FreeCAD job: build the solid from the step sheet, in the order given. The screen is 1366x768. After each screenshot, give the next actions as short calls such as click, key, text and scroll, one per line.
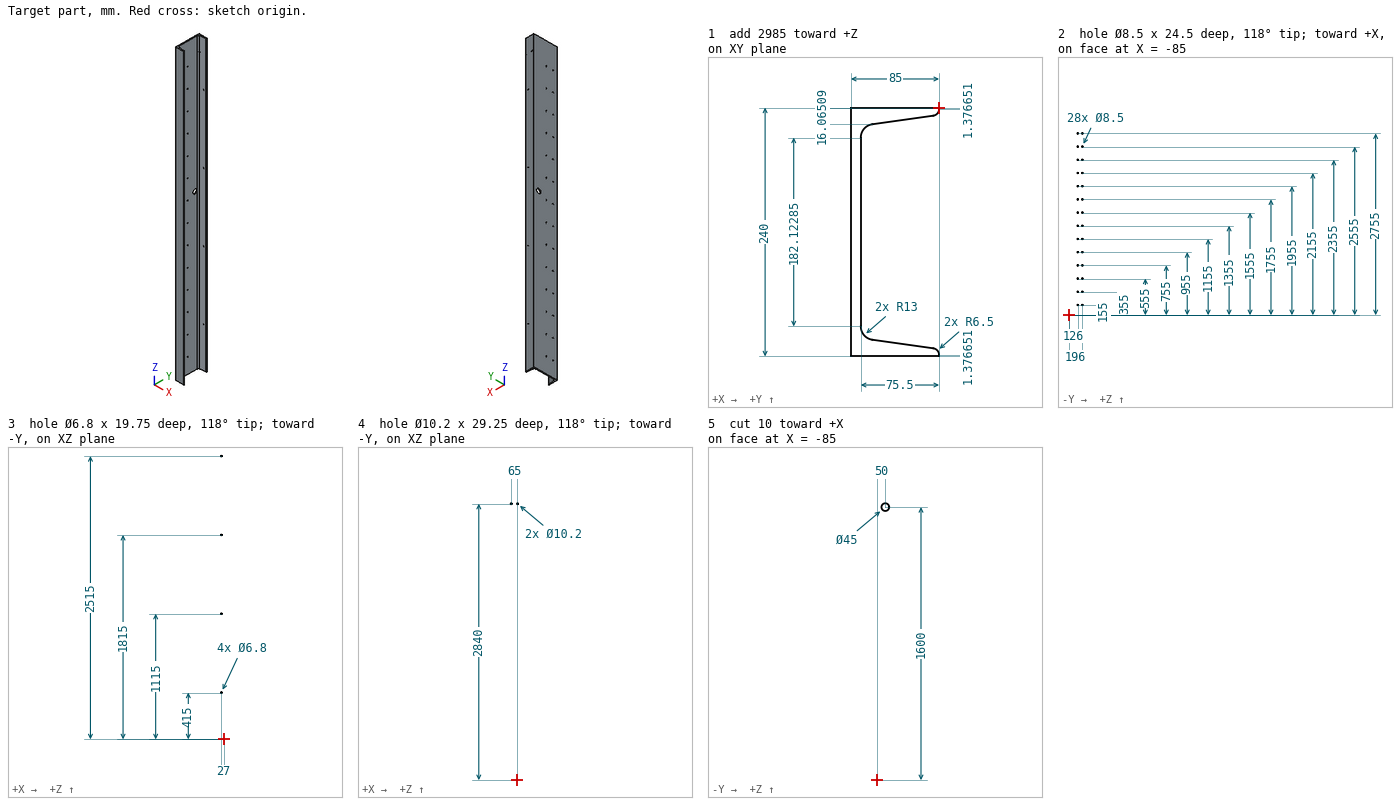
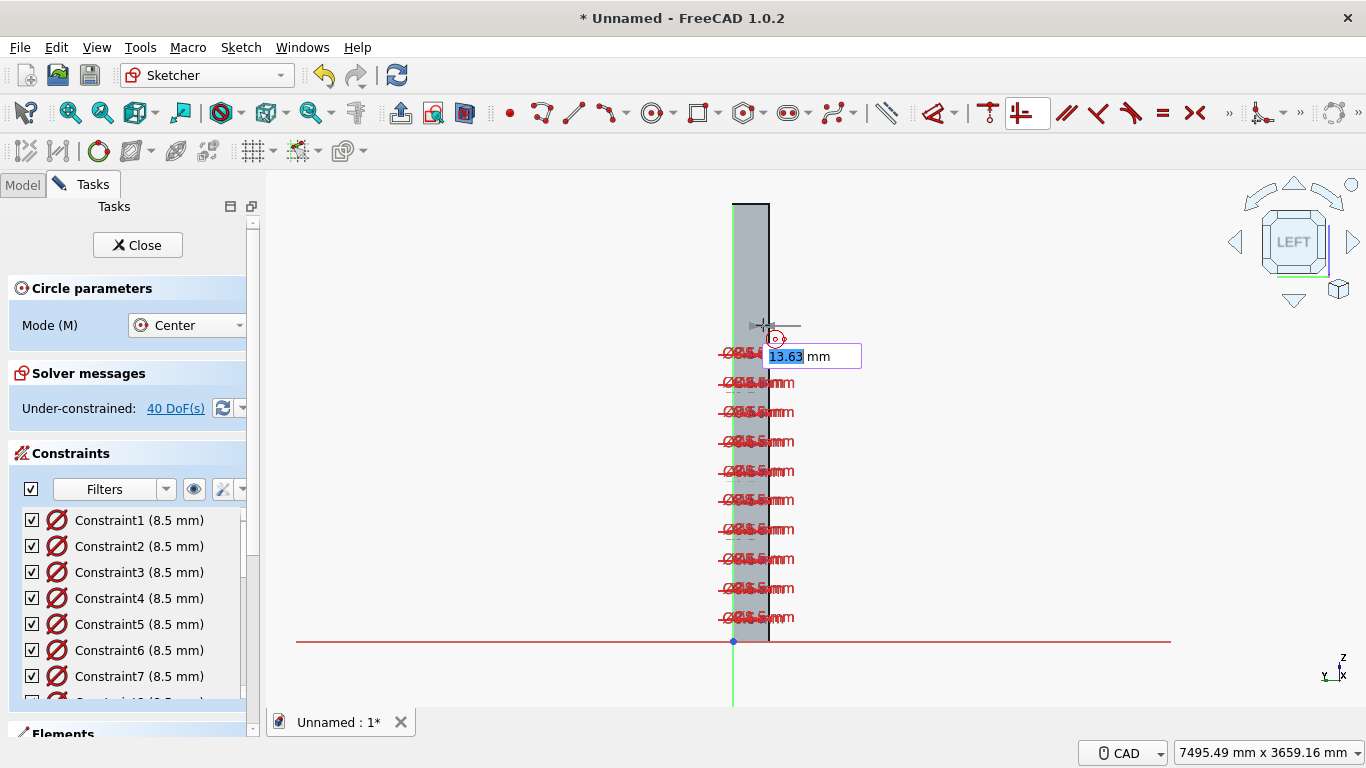
text(8.5)
key(Return)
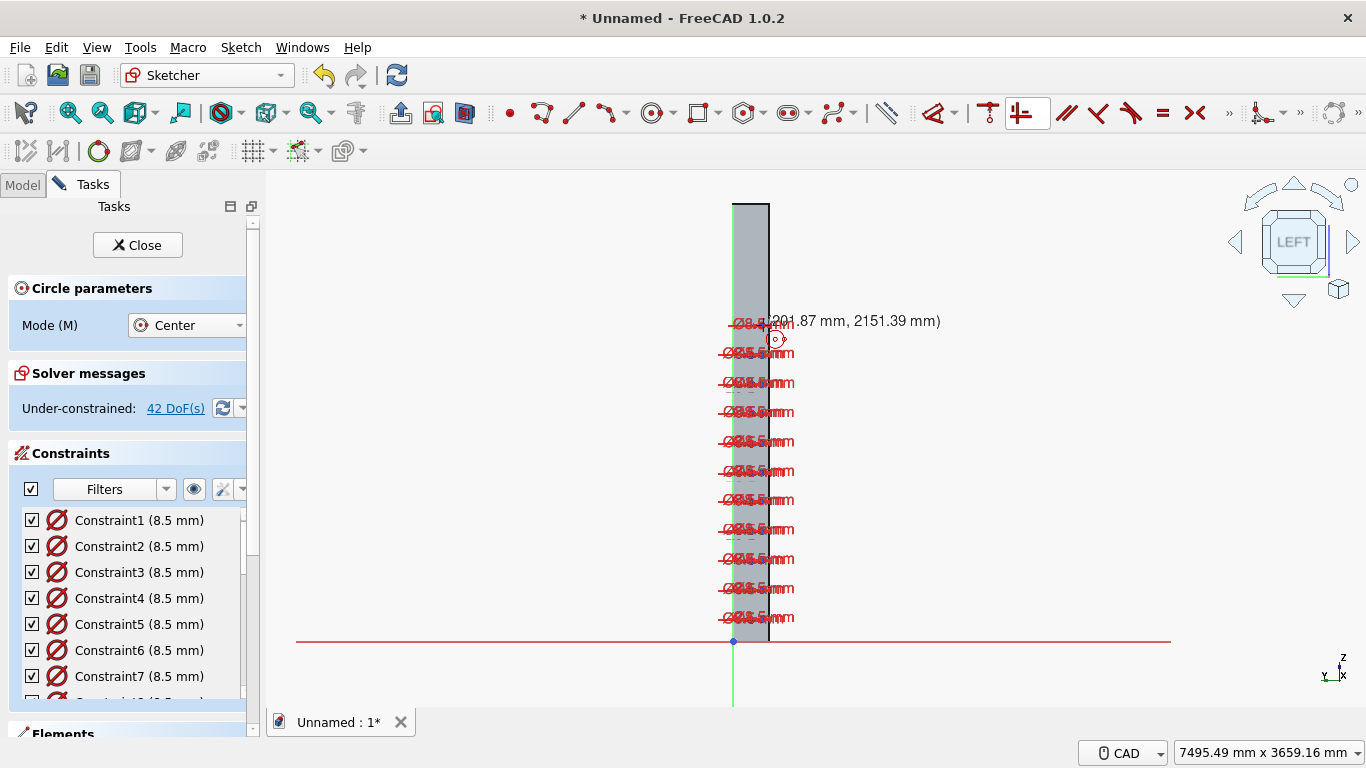
scroll(752, 325, up, 18)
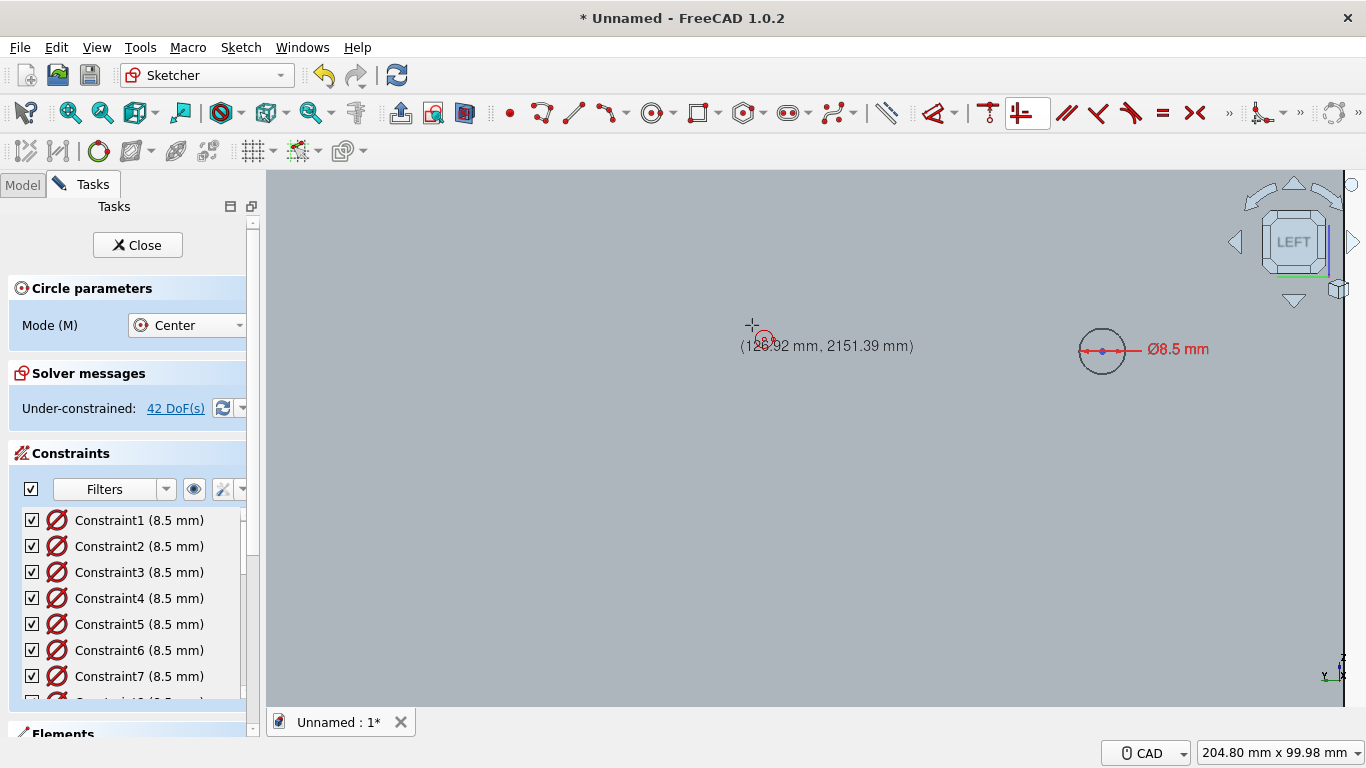
scroll(752, 325, down, 18)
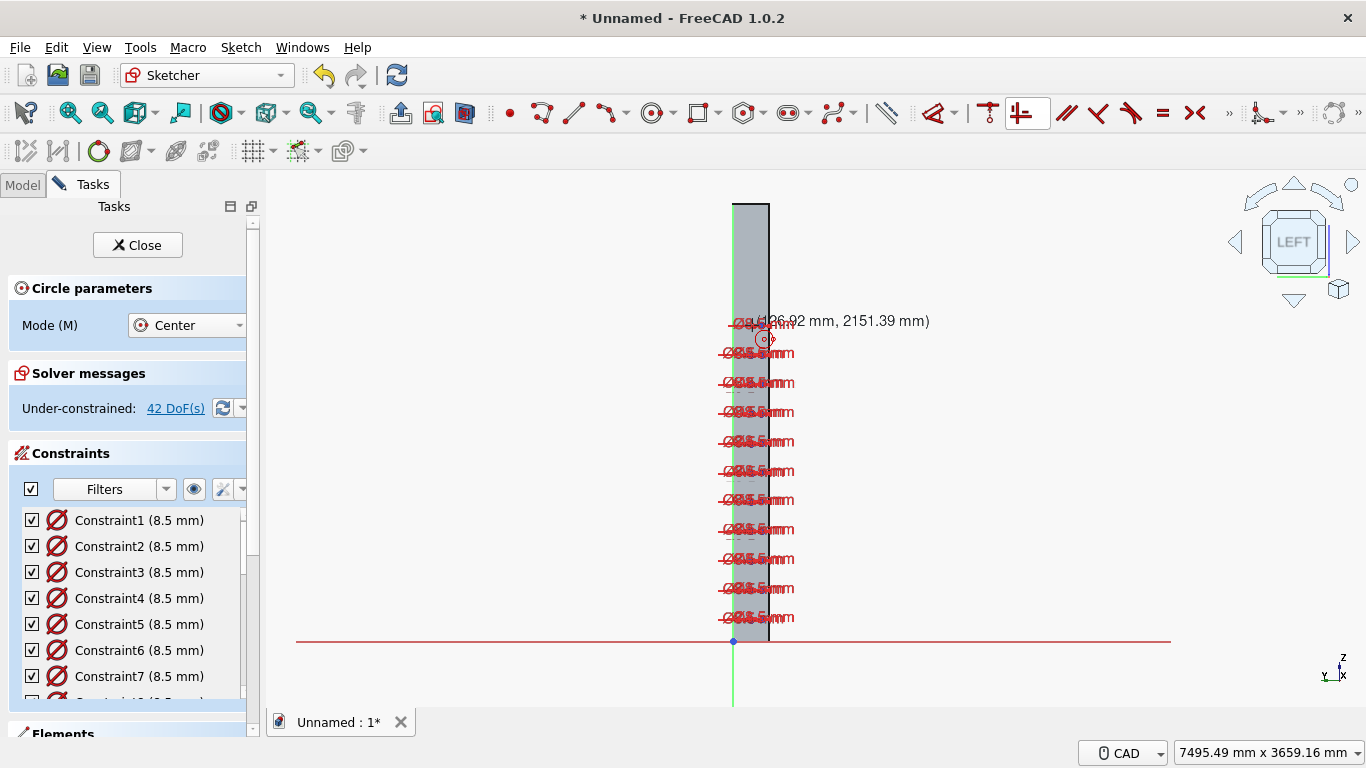
scroll(752, 325, up, 3)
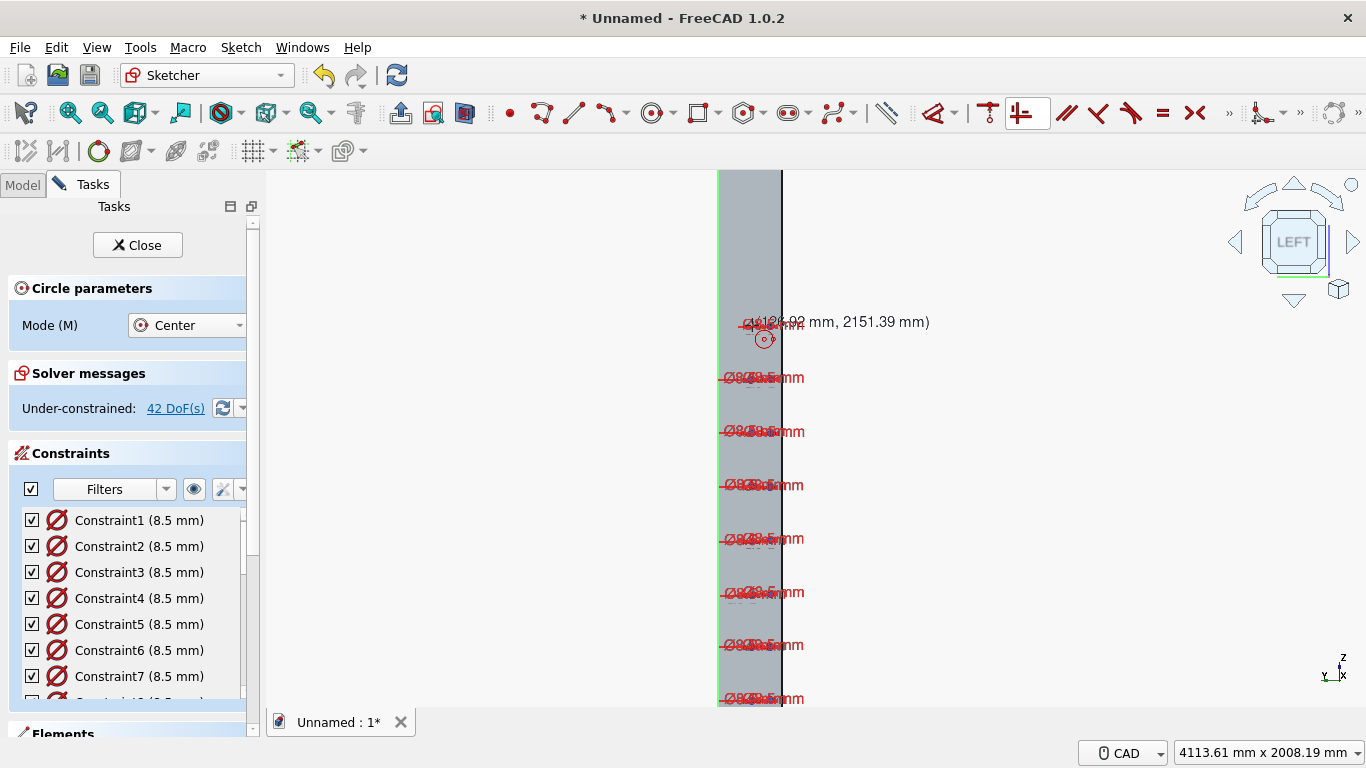
click(751, 326)
move(752, 325)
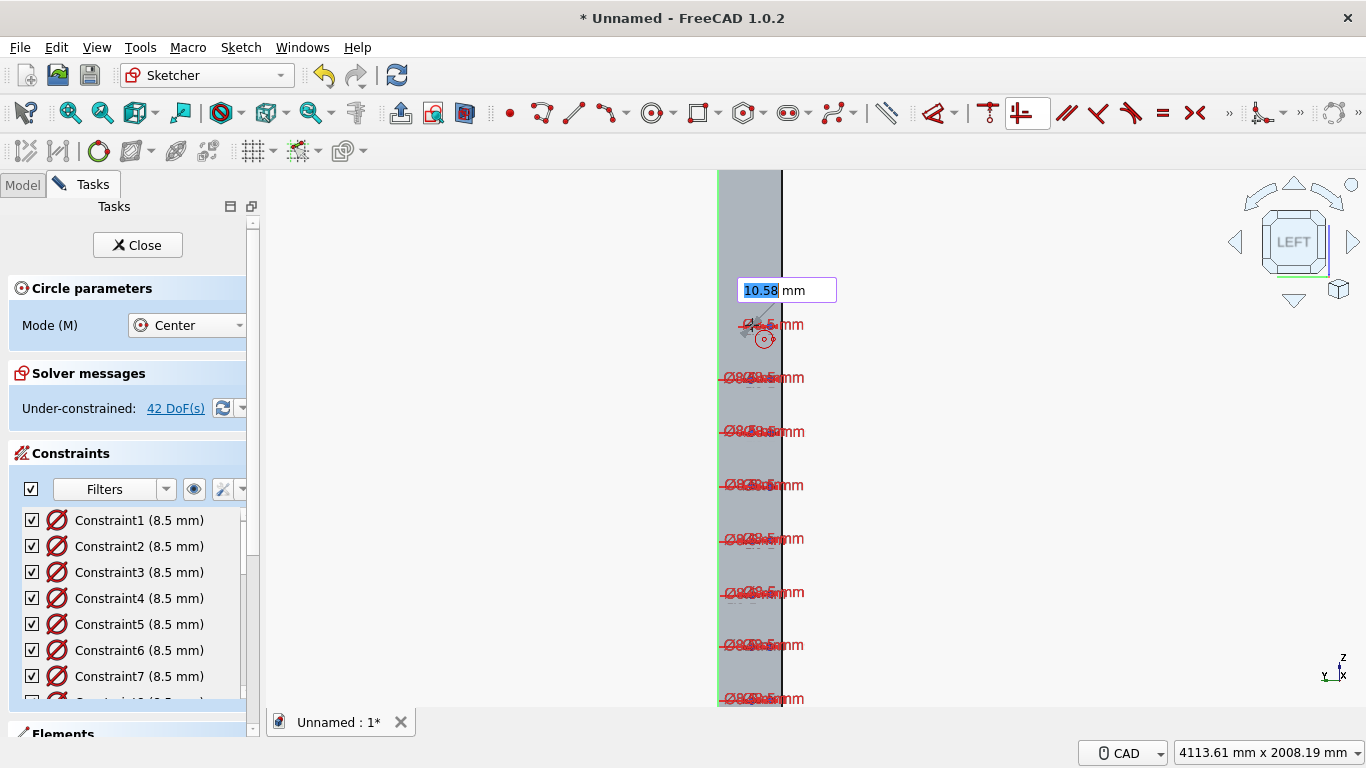
text(8.5)
key(Return)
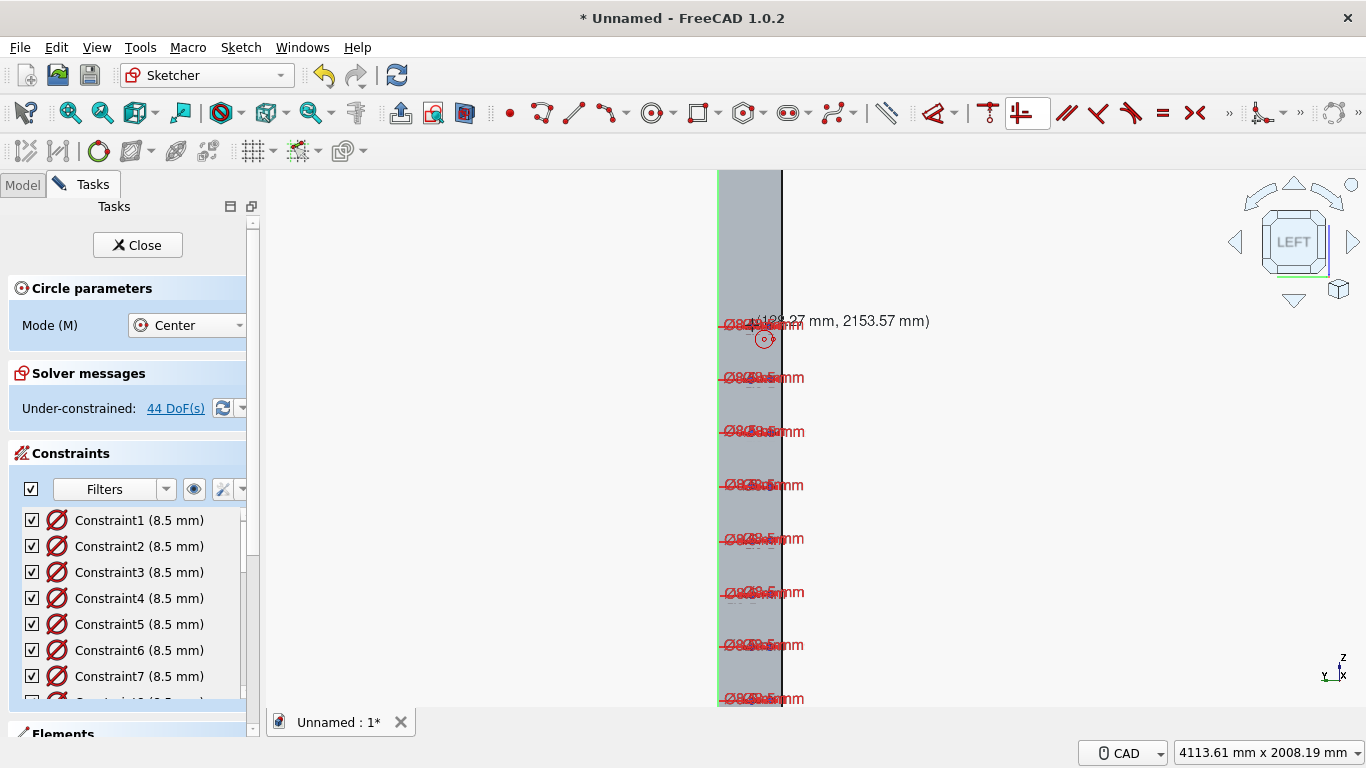
scroll(751, 272, up, 15)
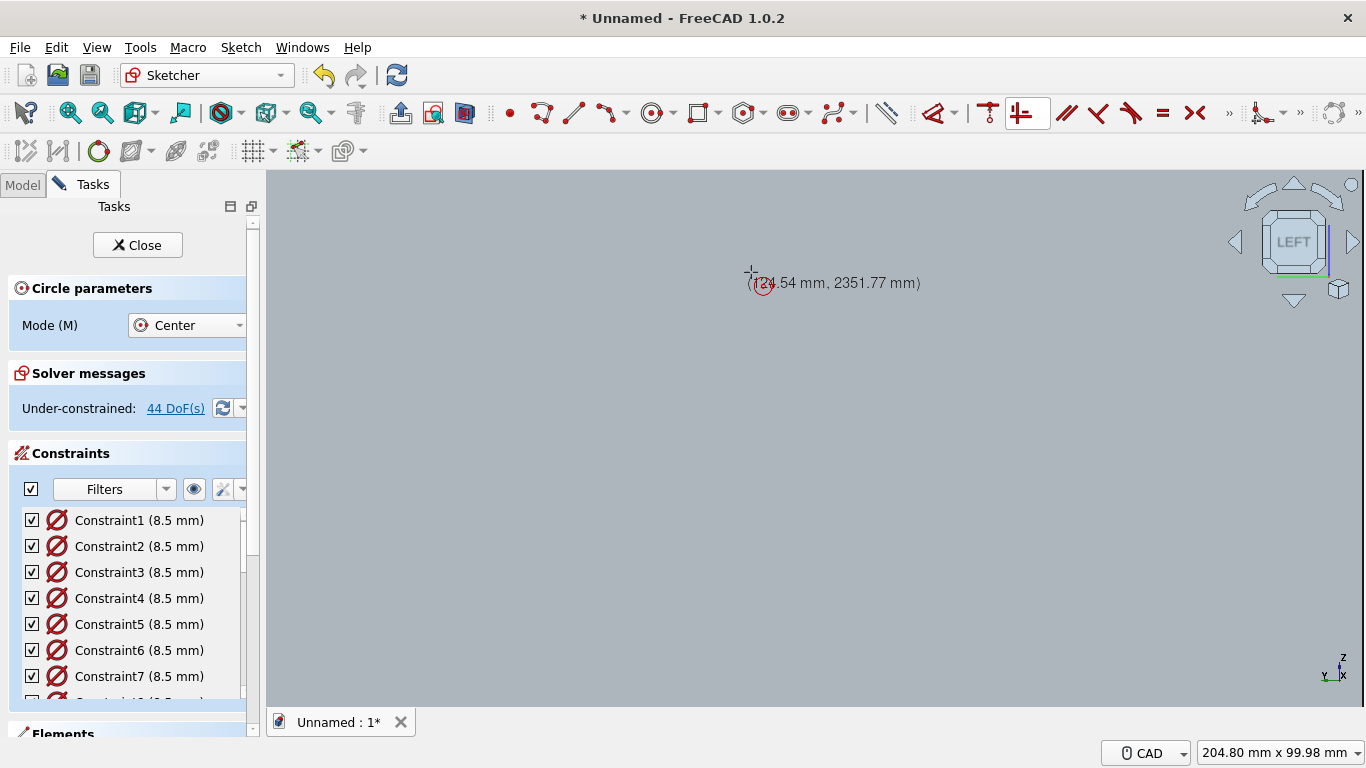
scroll(751, 296, down, 18)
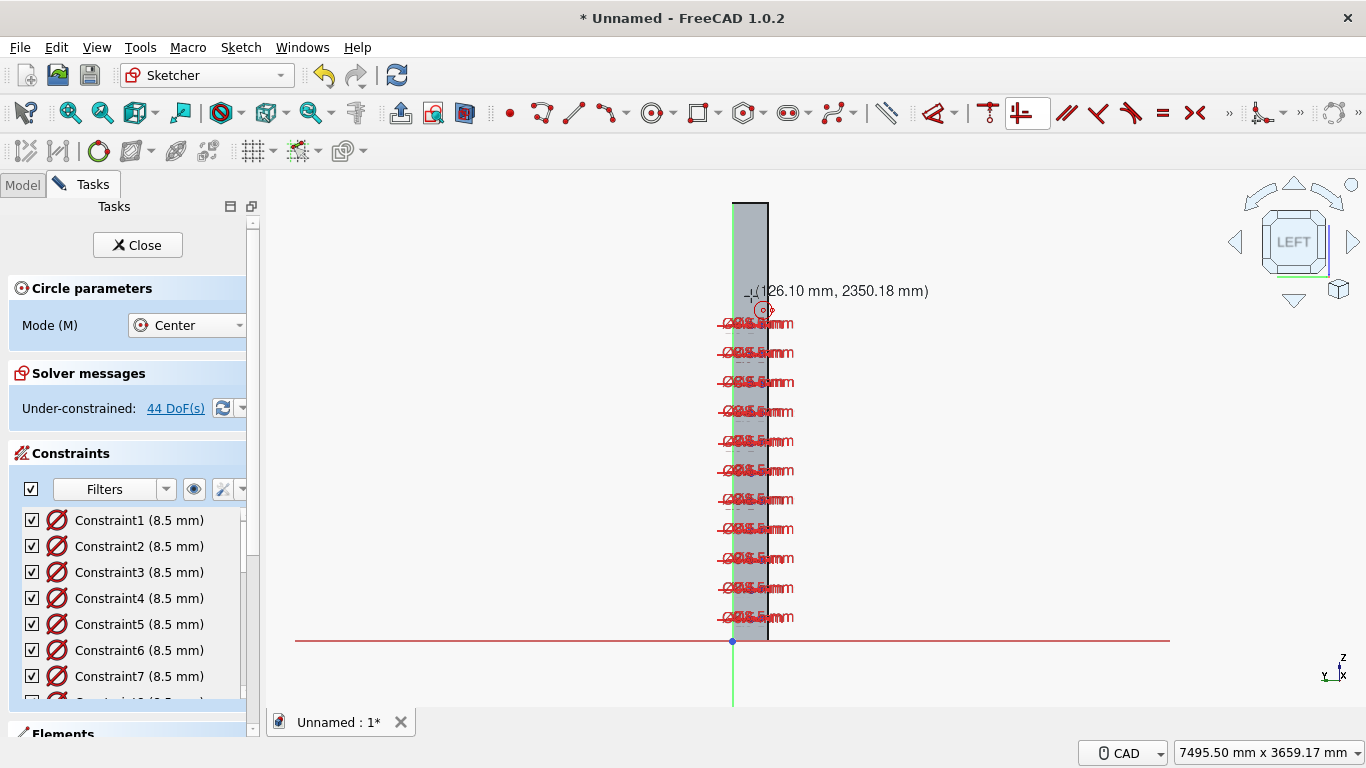
click(751, 296)
move(752, 295)